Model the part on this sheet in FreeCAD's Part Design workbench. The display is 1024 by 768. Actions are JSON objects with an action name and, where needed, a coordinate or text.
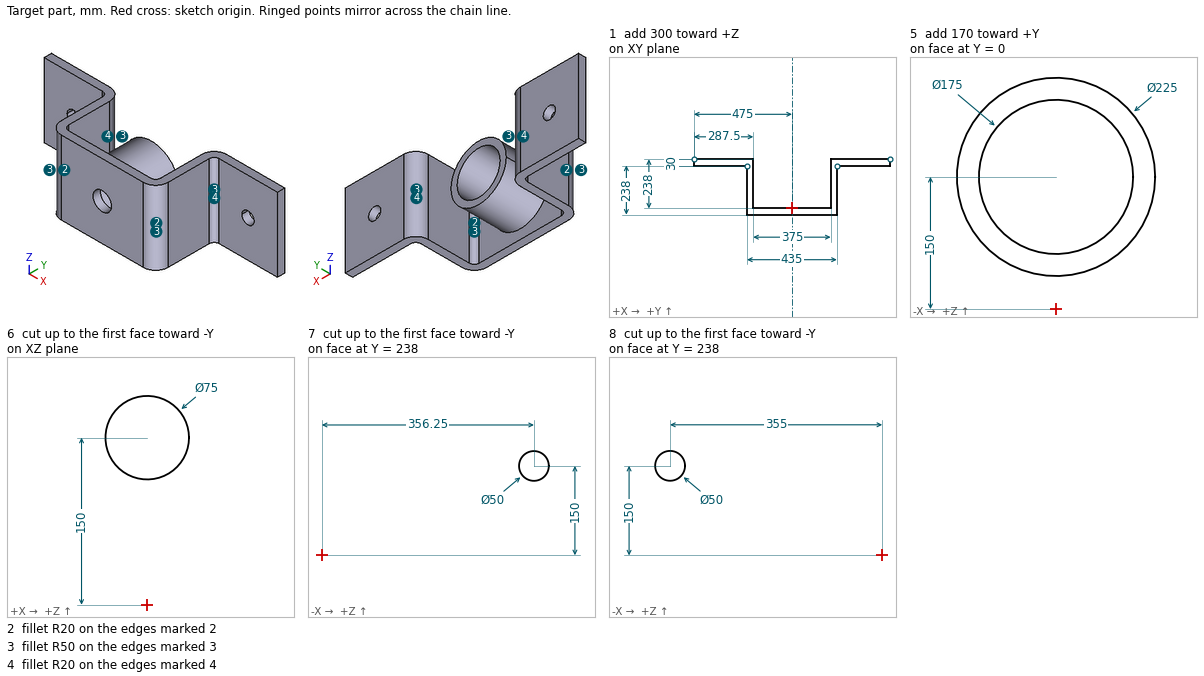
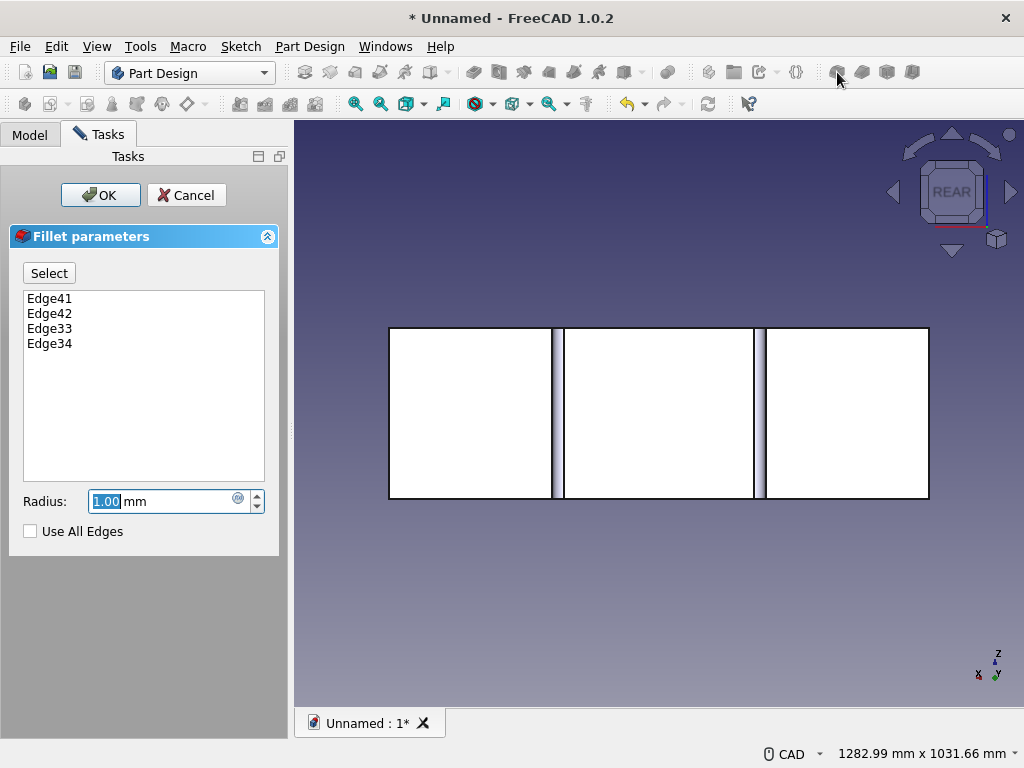
{"action": "type", "text": "50"}
{"action": "key", "text": "Tab"}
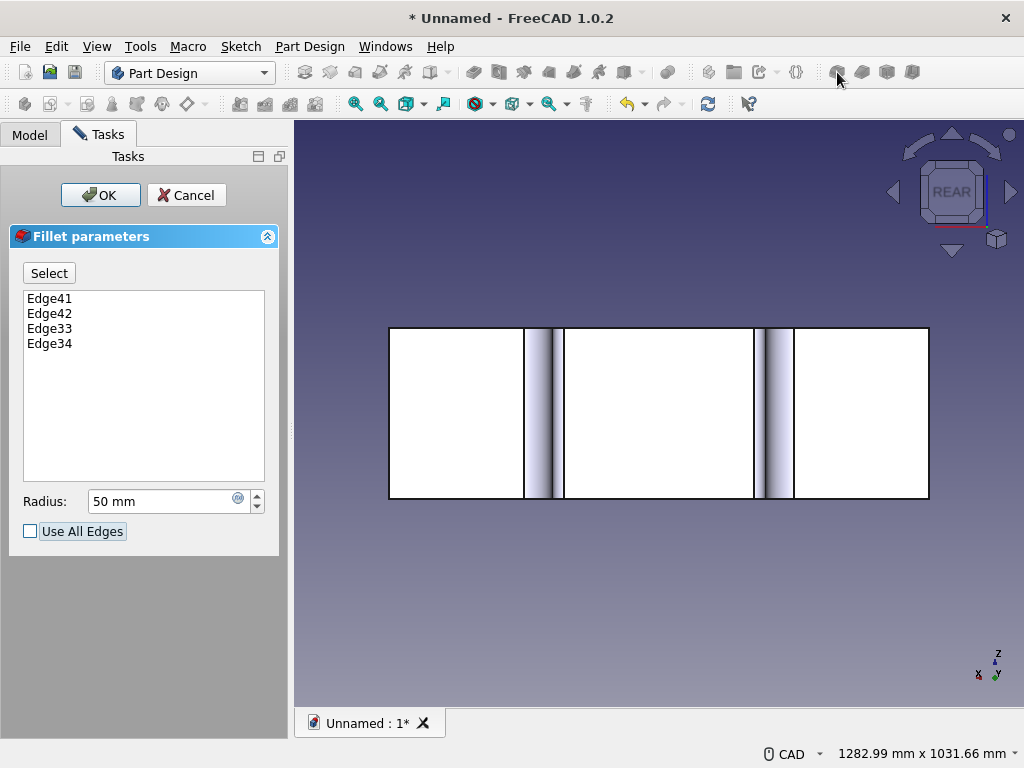
{"action": "left_click", "coordinate": [101, 195]}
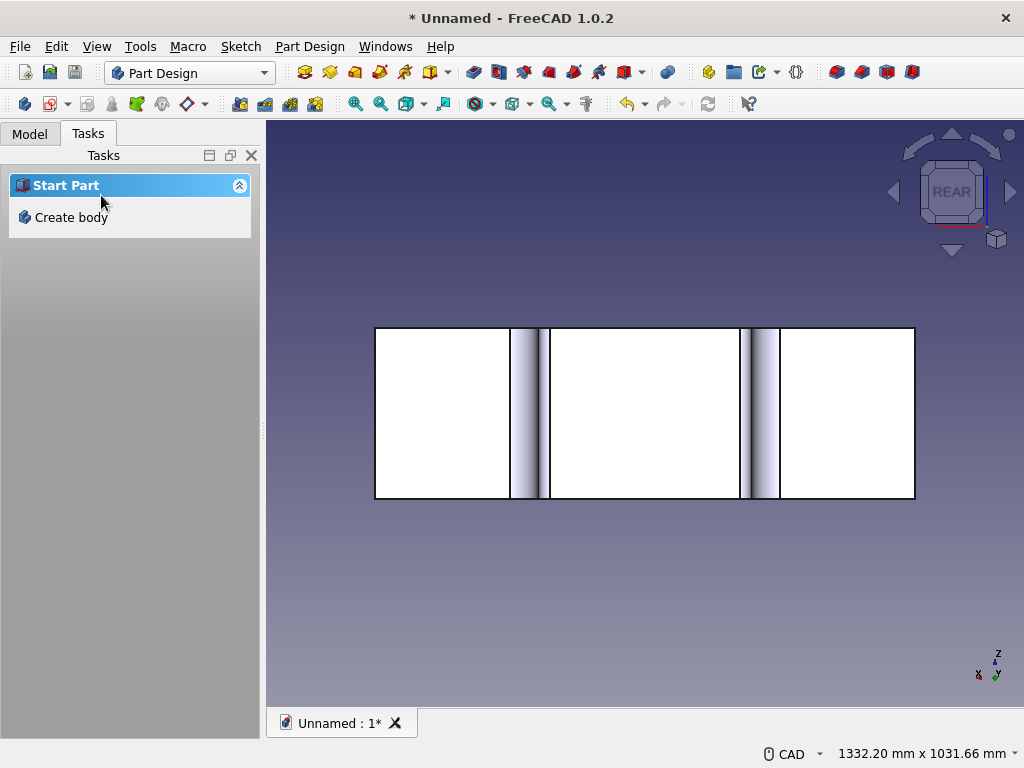
{"action": "key", "text": "0"}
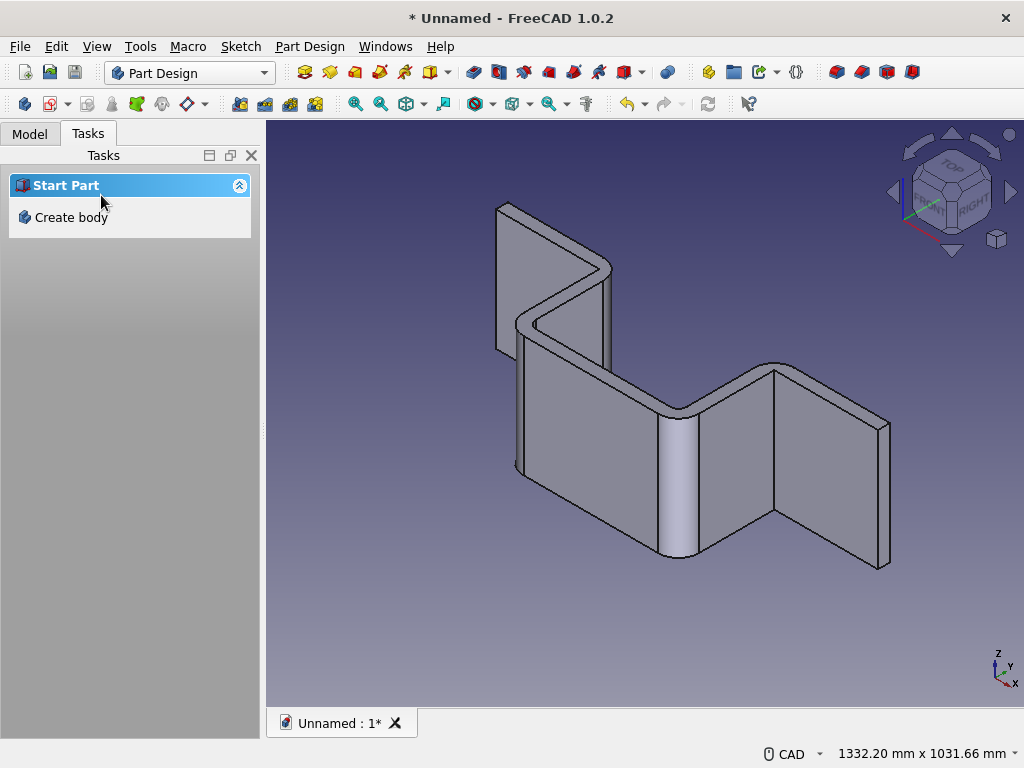
{"action": "key", "text": "2"}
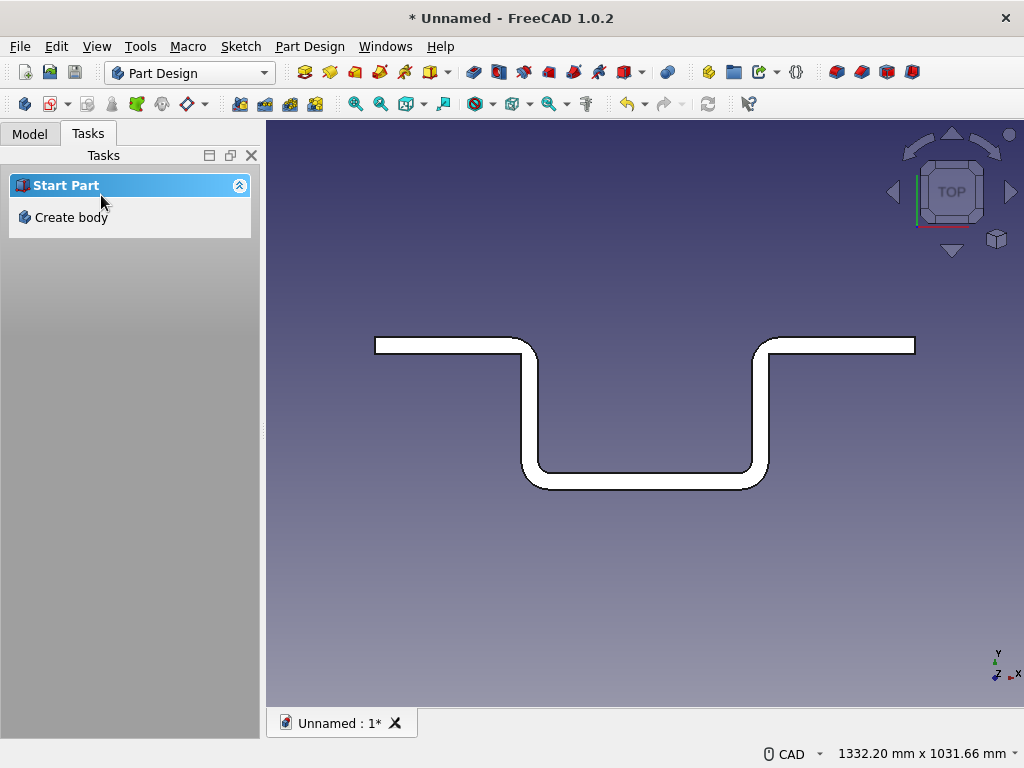
{"action": "key", "text": "1"}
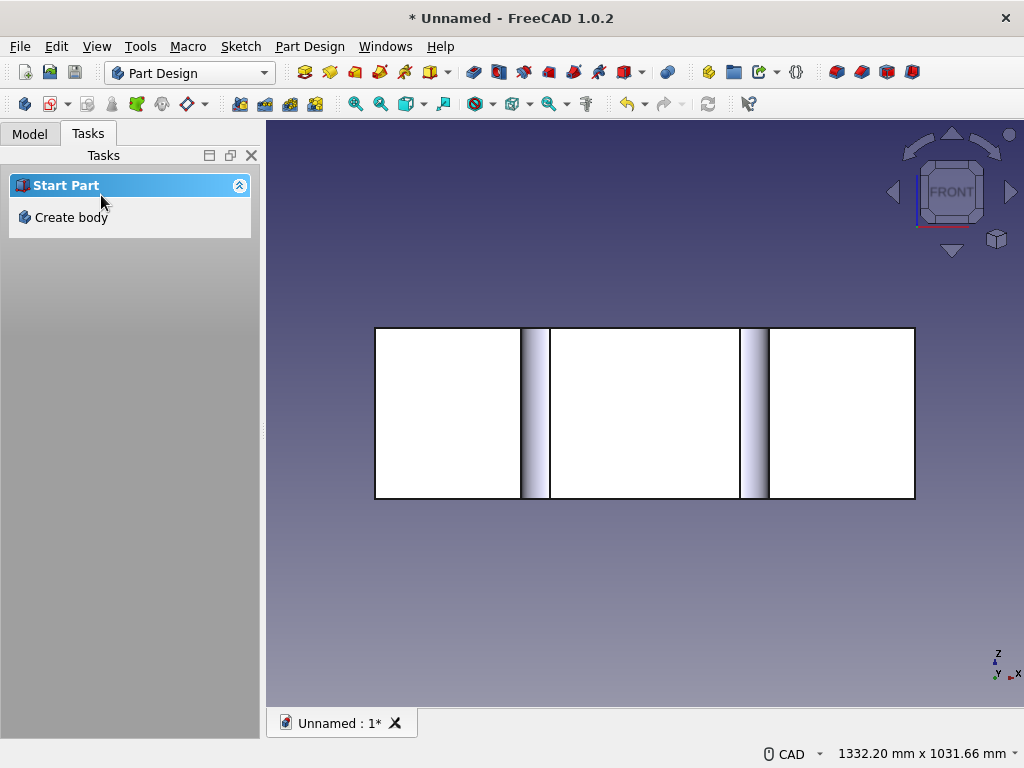
{"action": "key", "text": "3"}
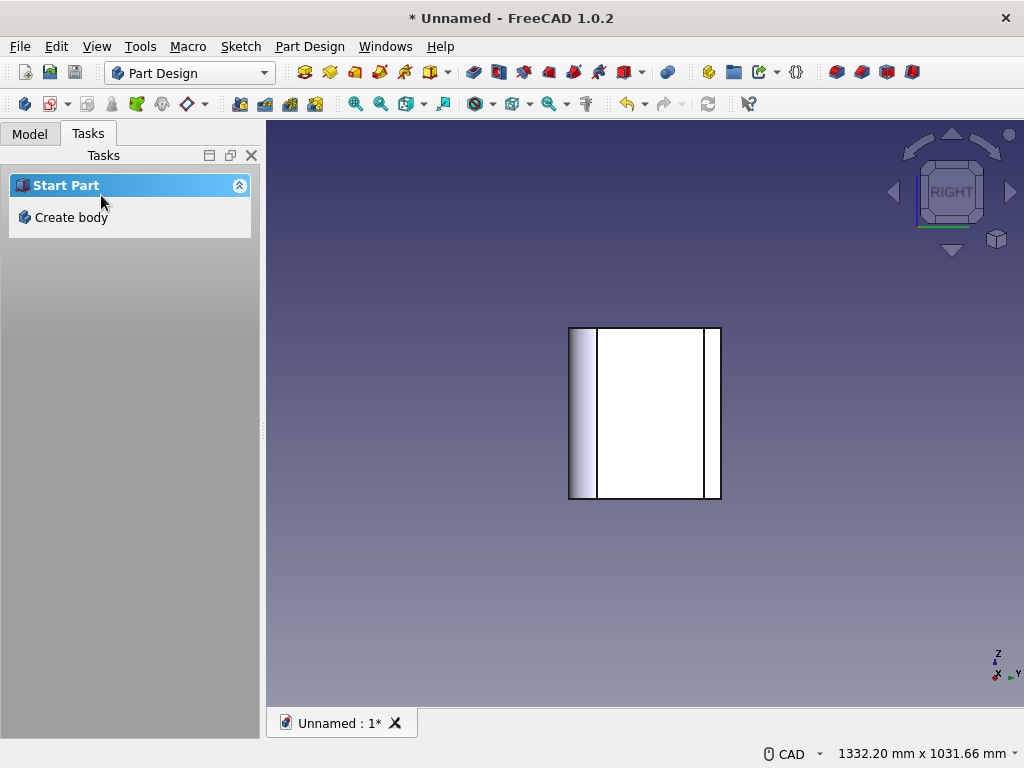
{"action": "left_click", "coordinate": [356, 104]}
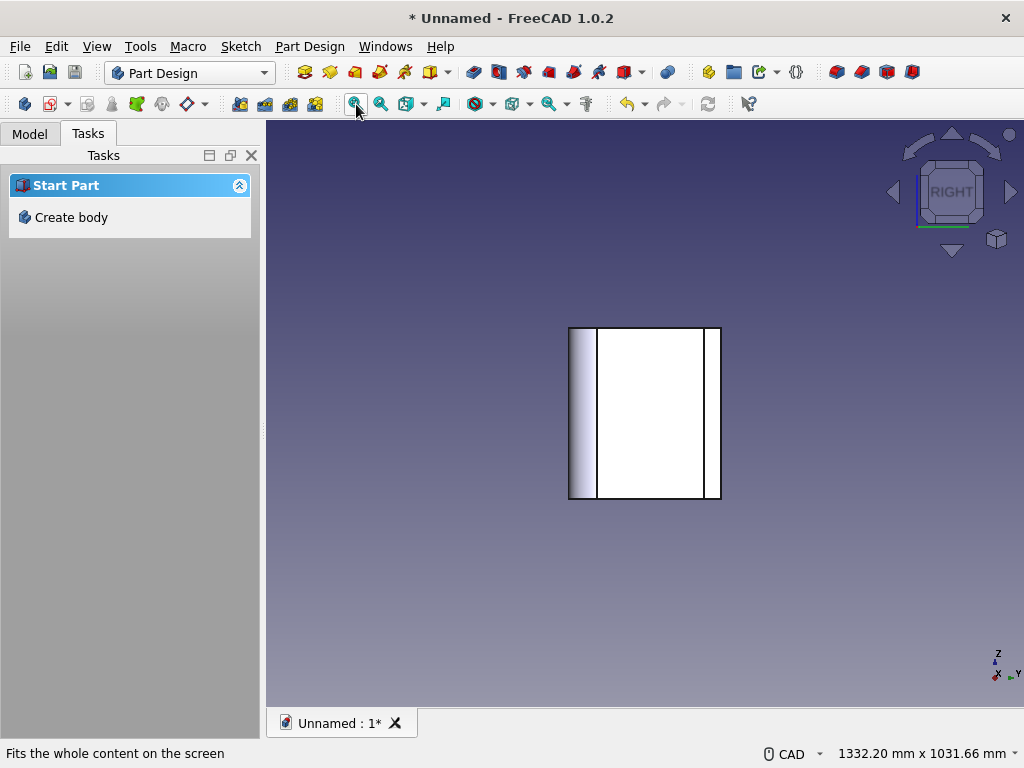
{"action": "key", "text": "5"}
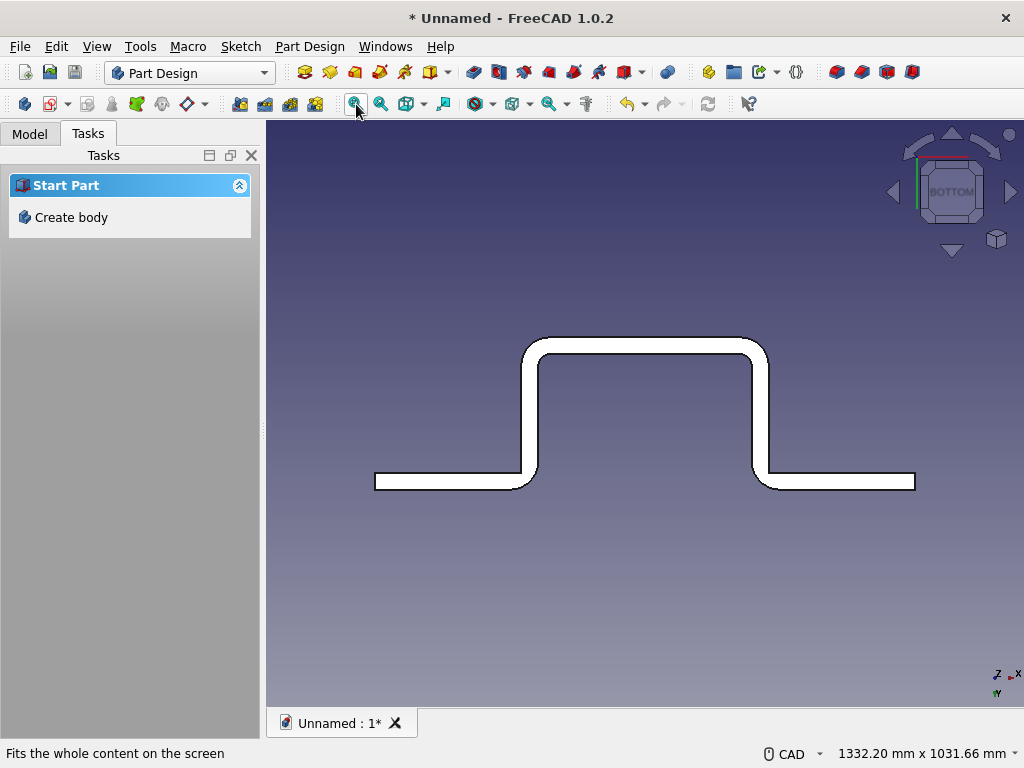
{"action": "key", "text": "4"}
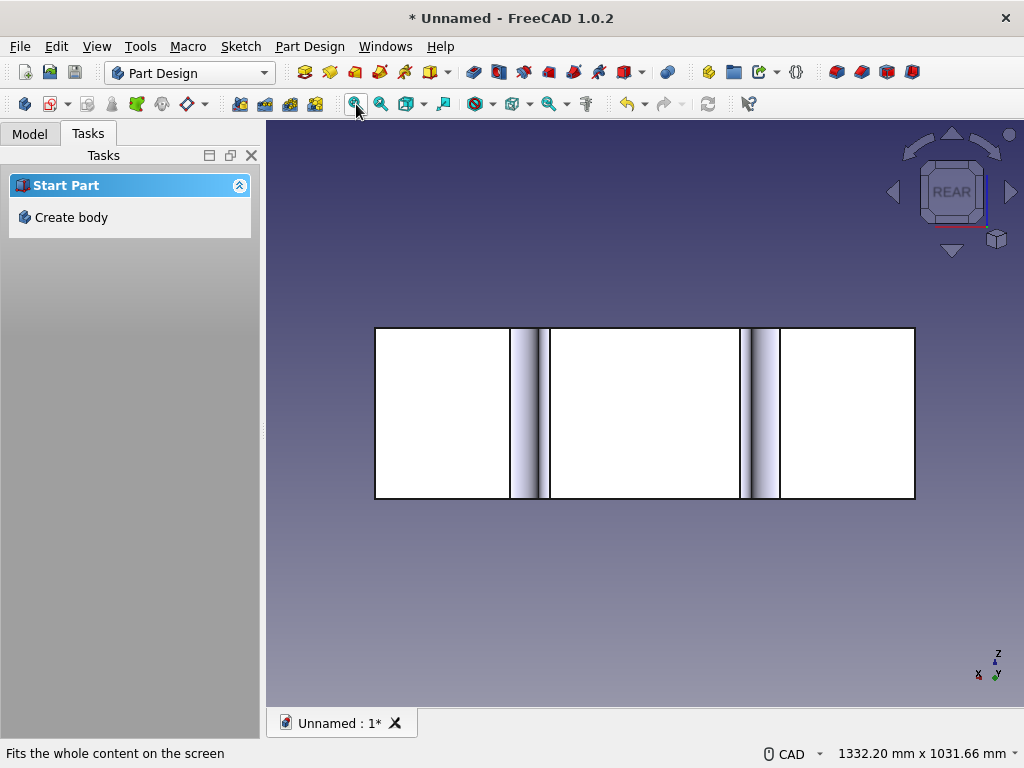
{"action": "key", "text": "6"}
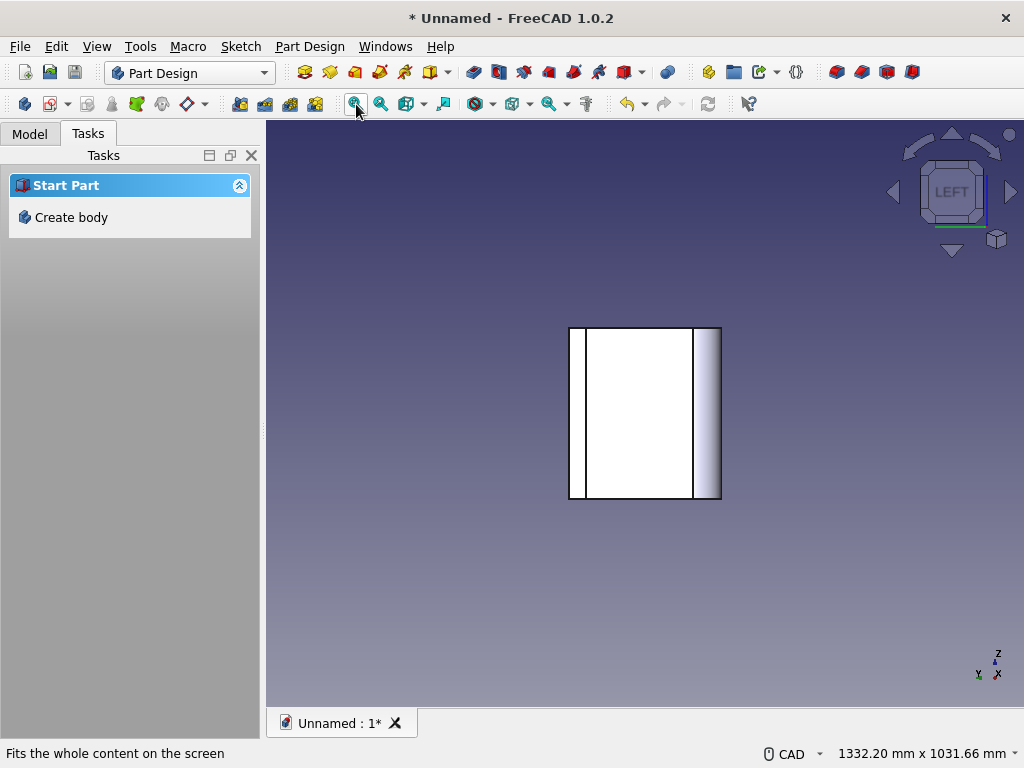
{"action": "left_click", "coordinate": [356, 104]}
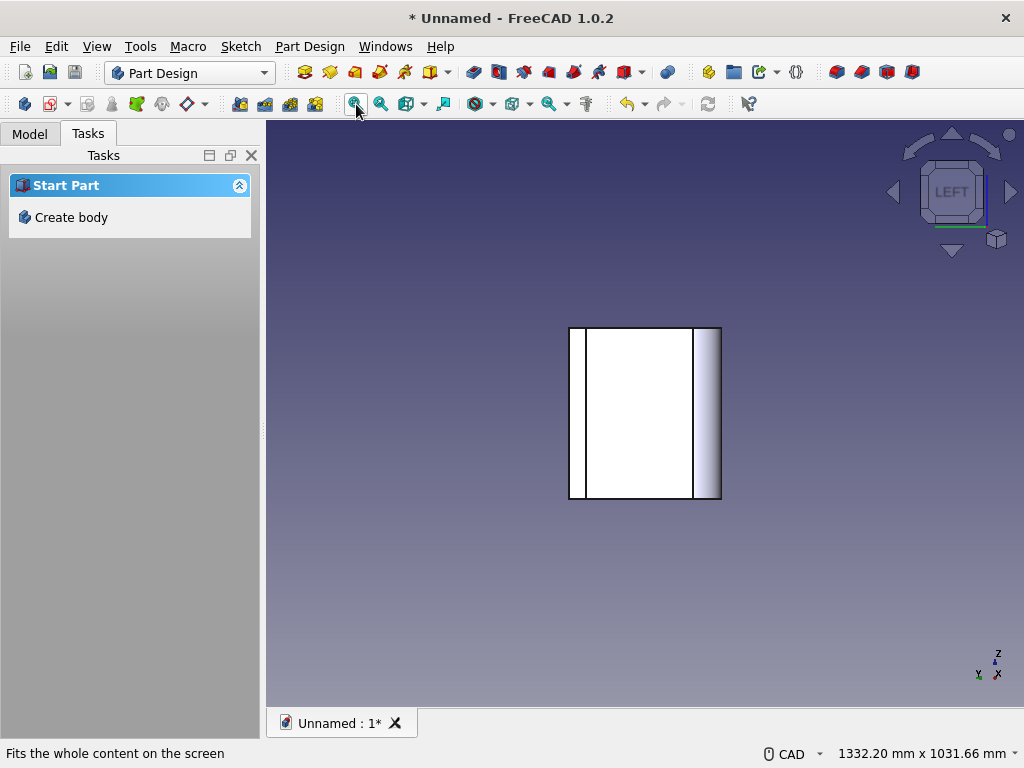
{"action": "key", "text": "v 3"}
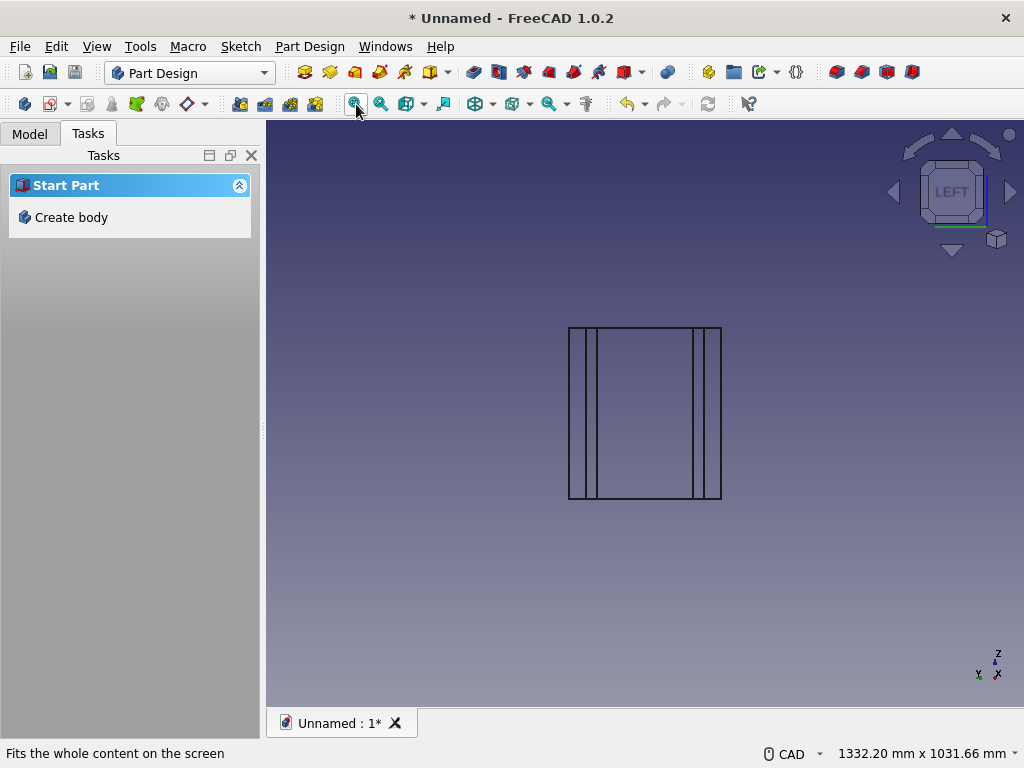
{"action": "key", "text": "0"}